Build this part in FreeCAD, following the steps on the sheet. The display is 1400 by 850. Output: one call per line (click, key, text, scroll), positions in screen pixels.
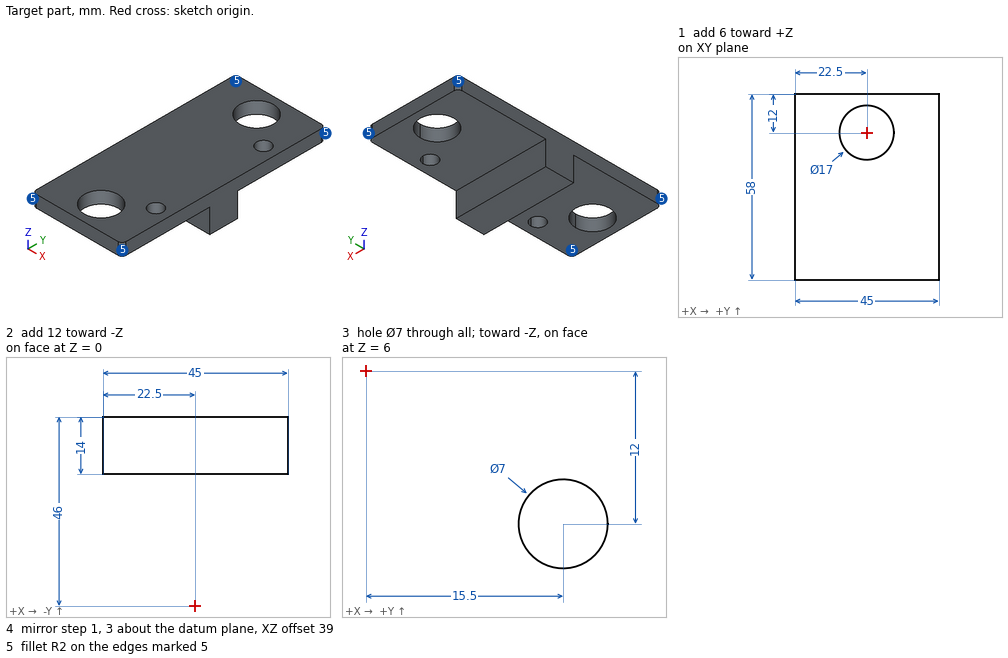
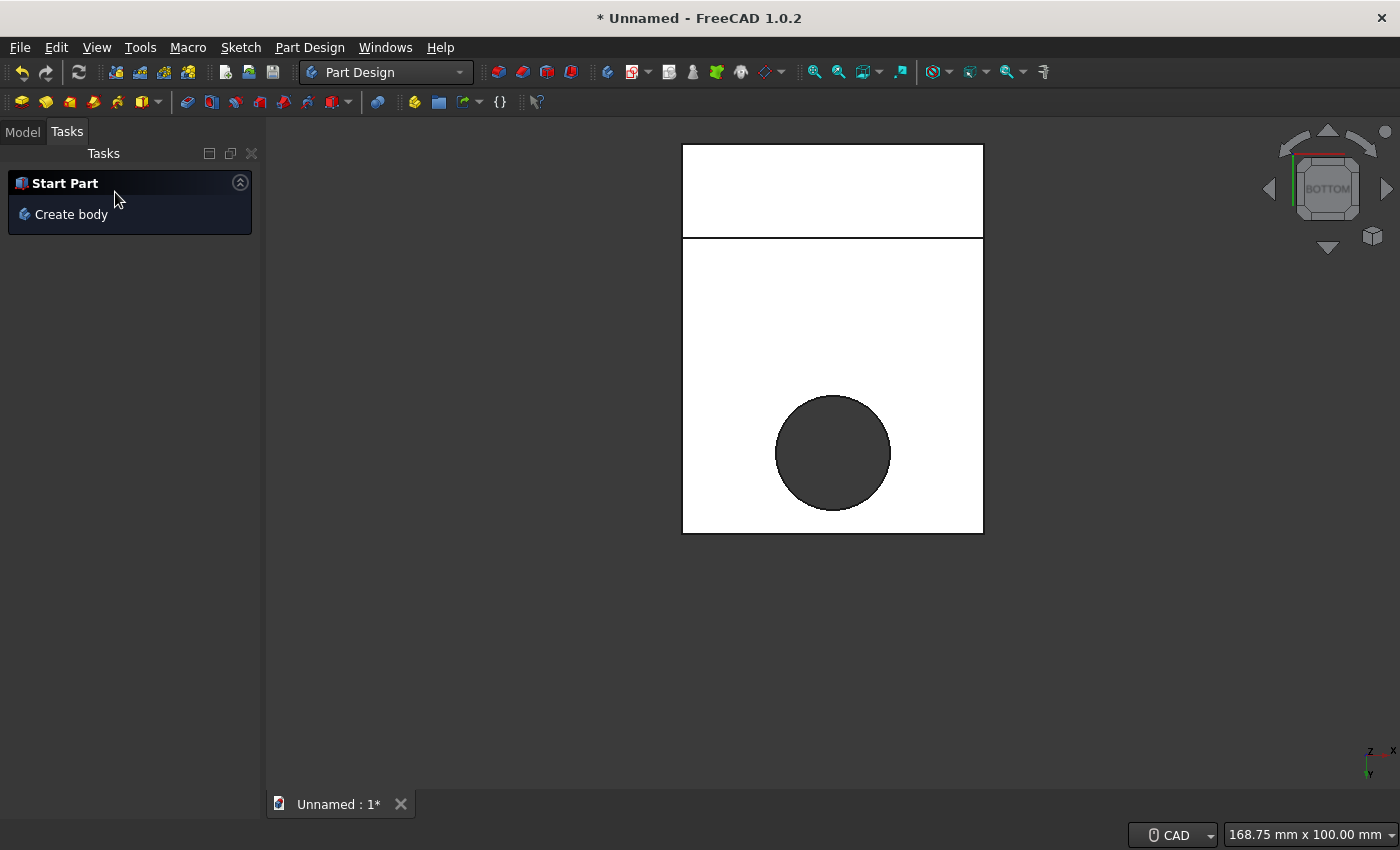
key(0)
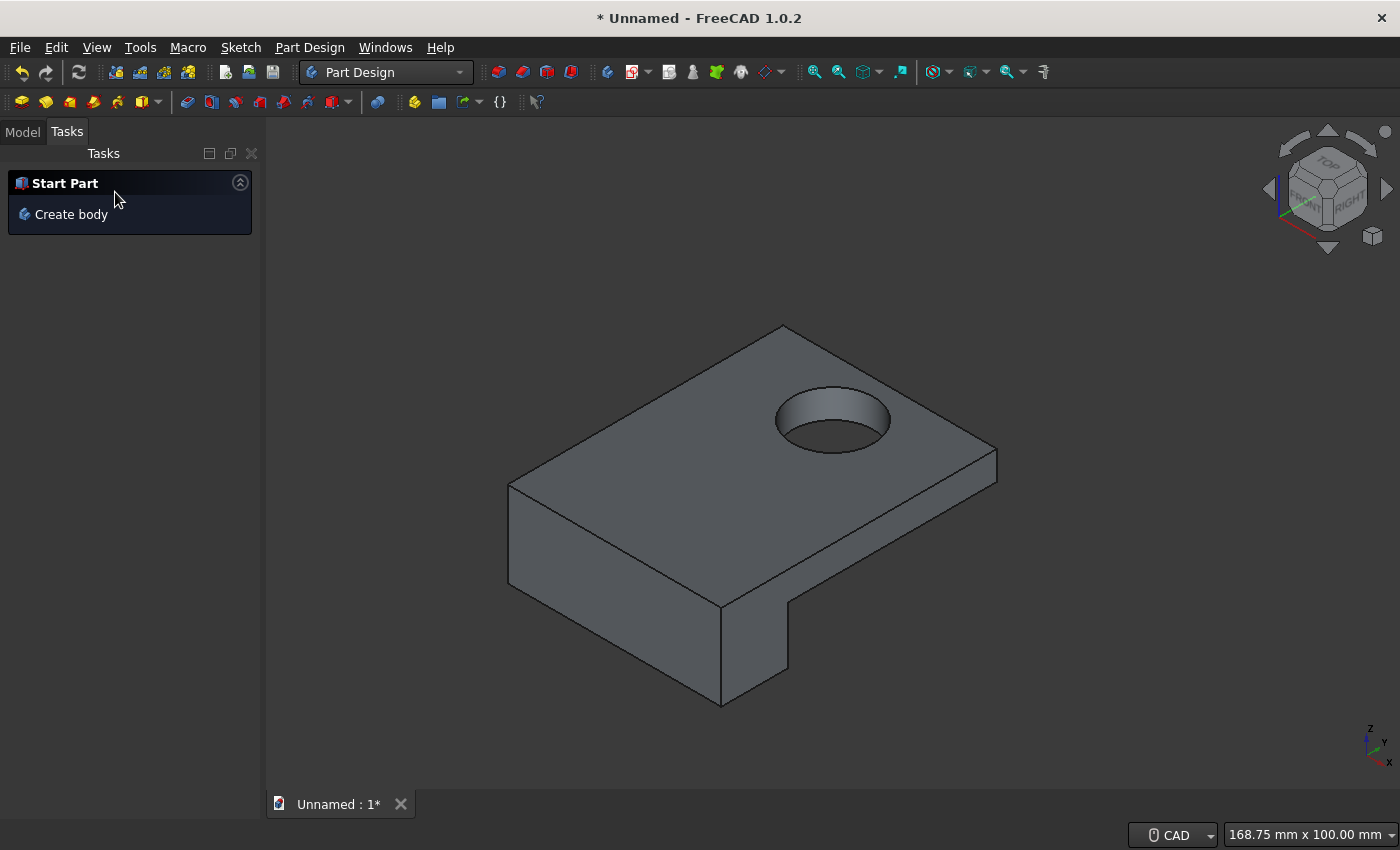
click(713, 488)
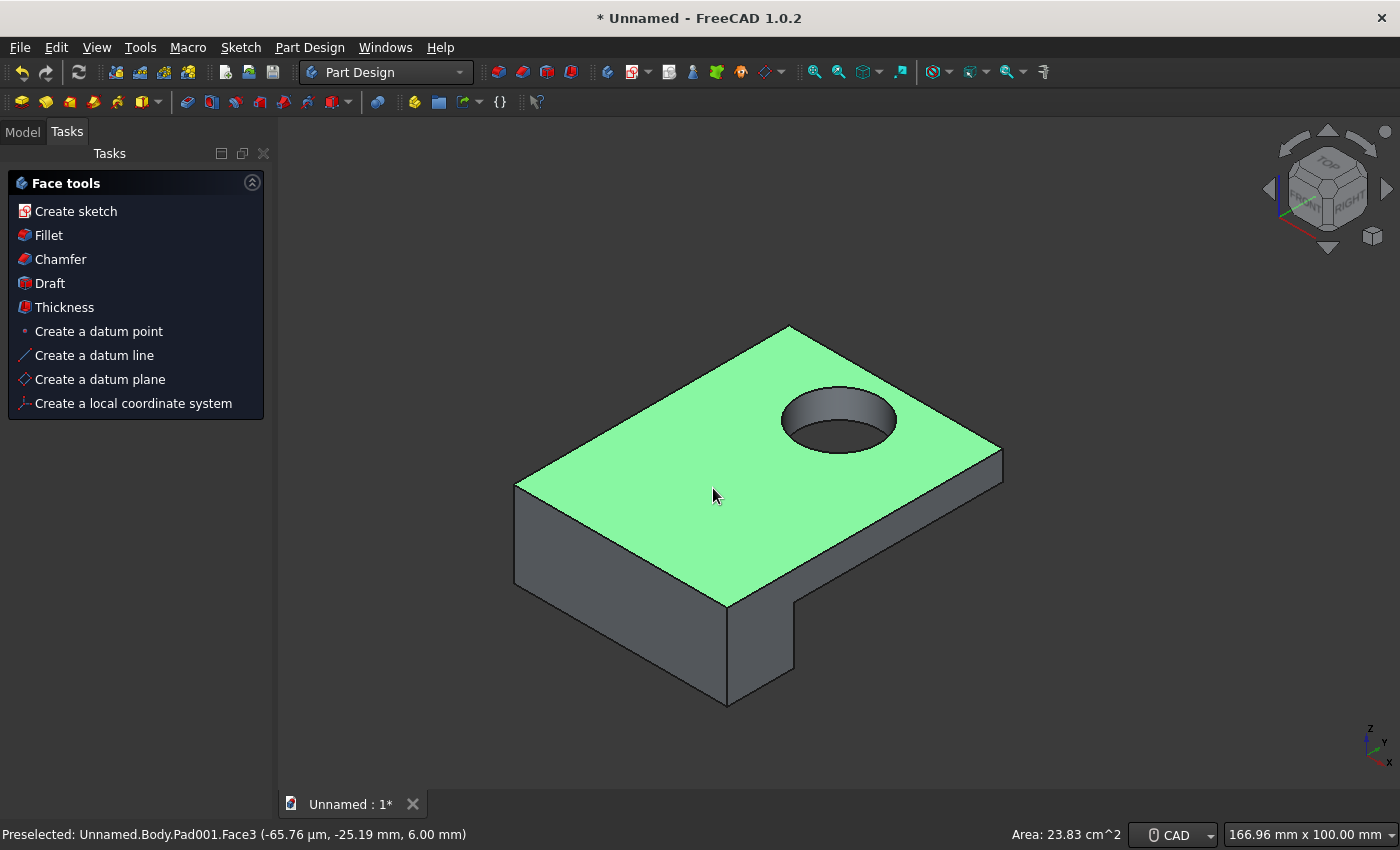
click(632, 72)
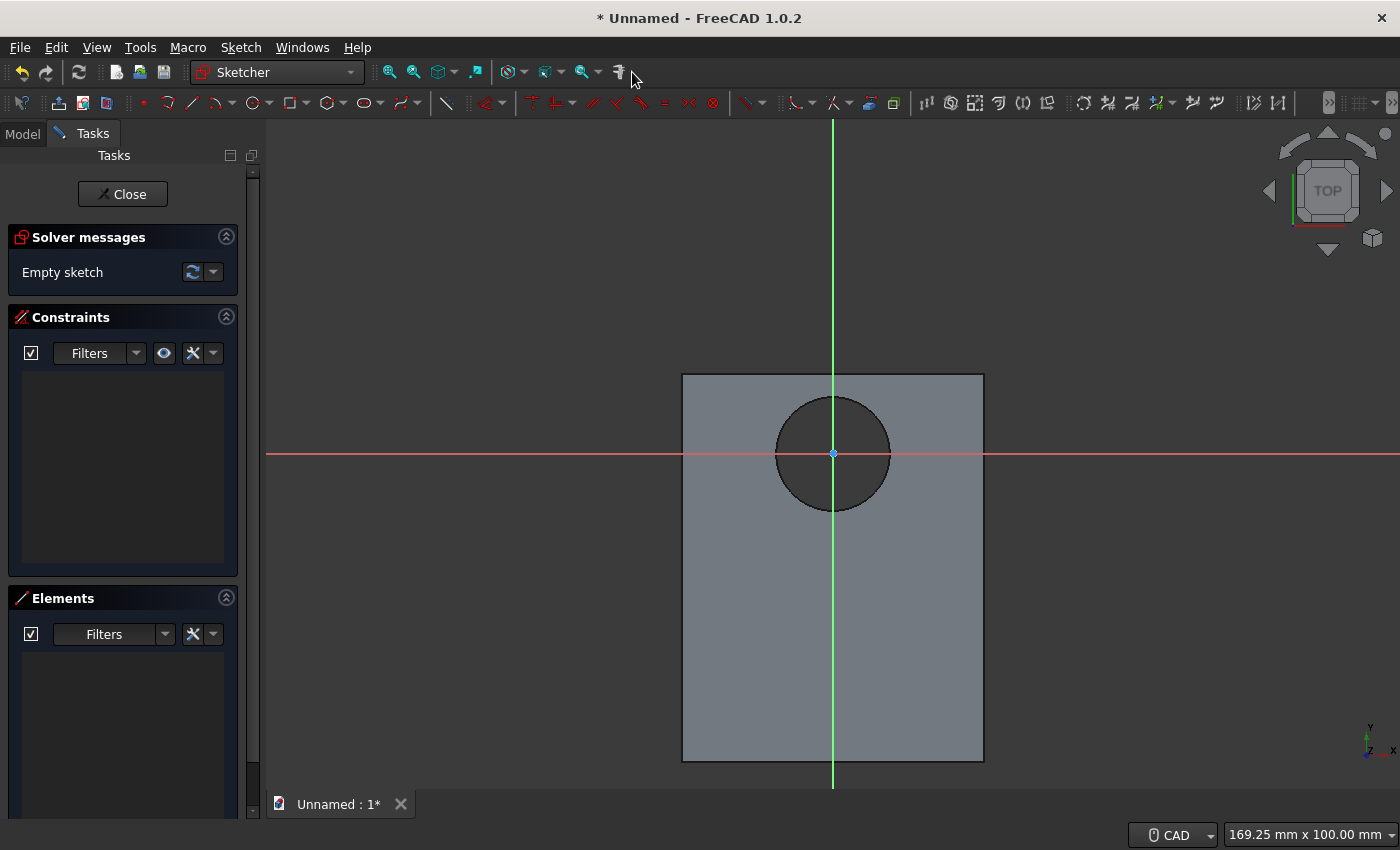
scroll(958, 544, up, 11)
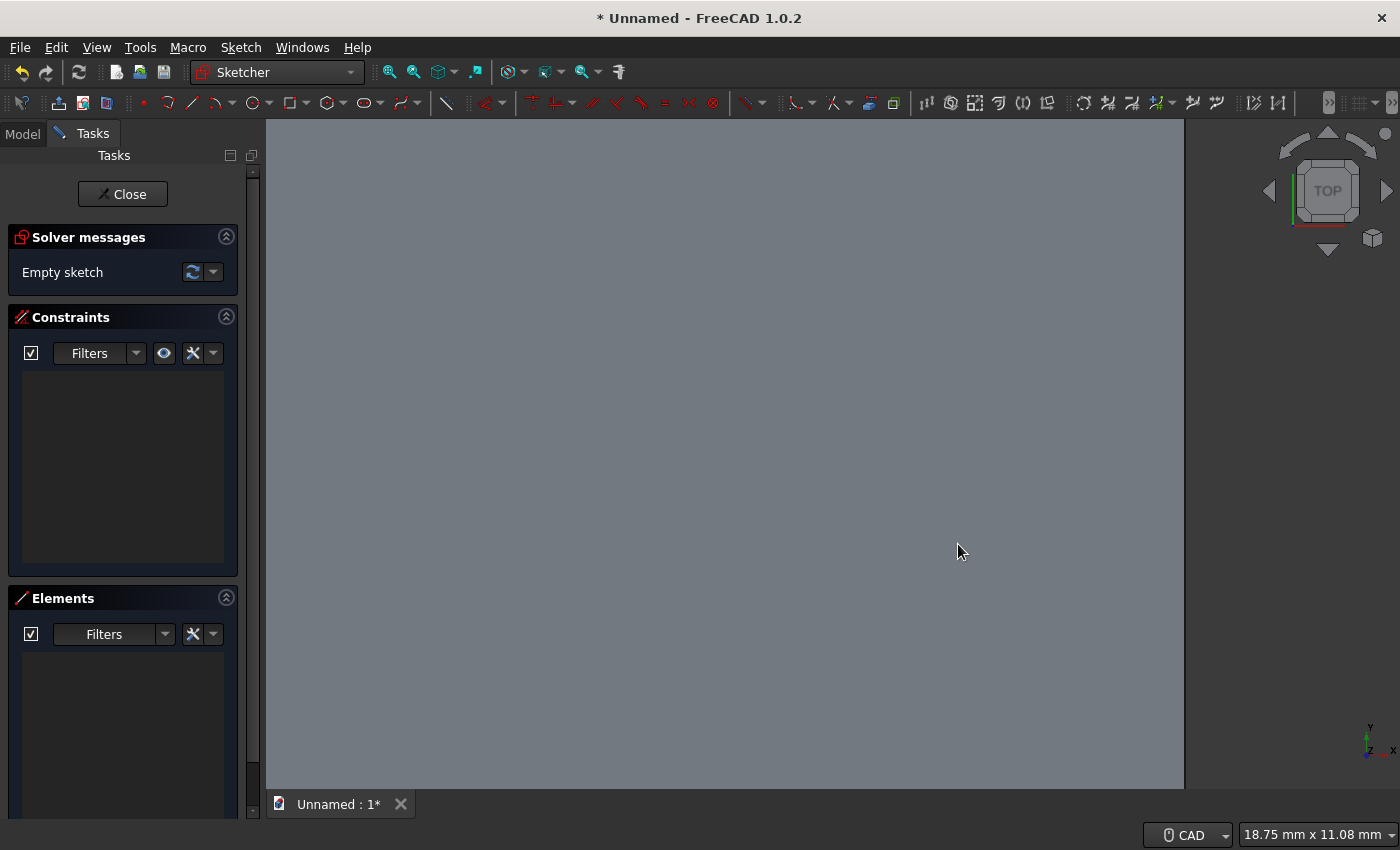
click(254, 104)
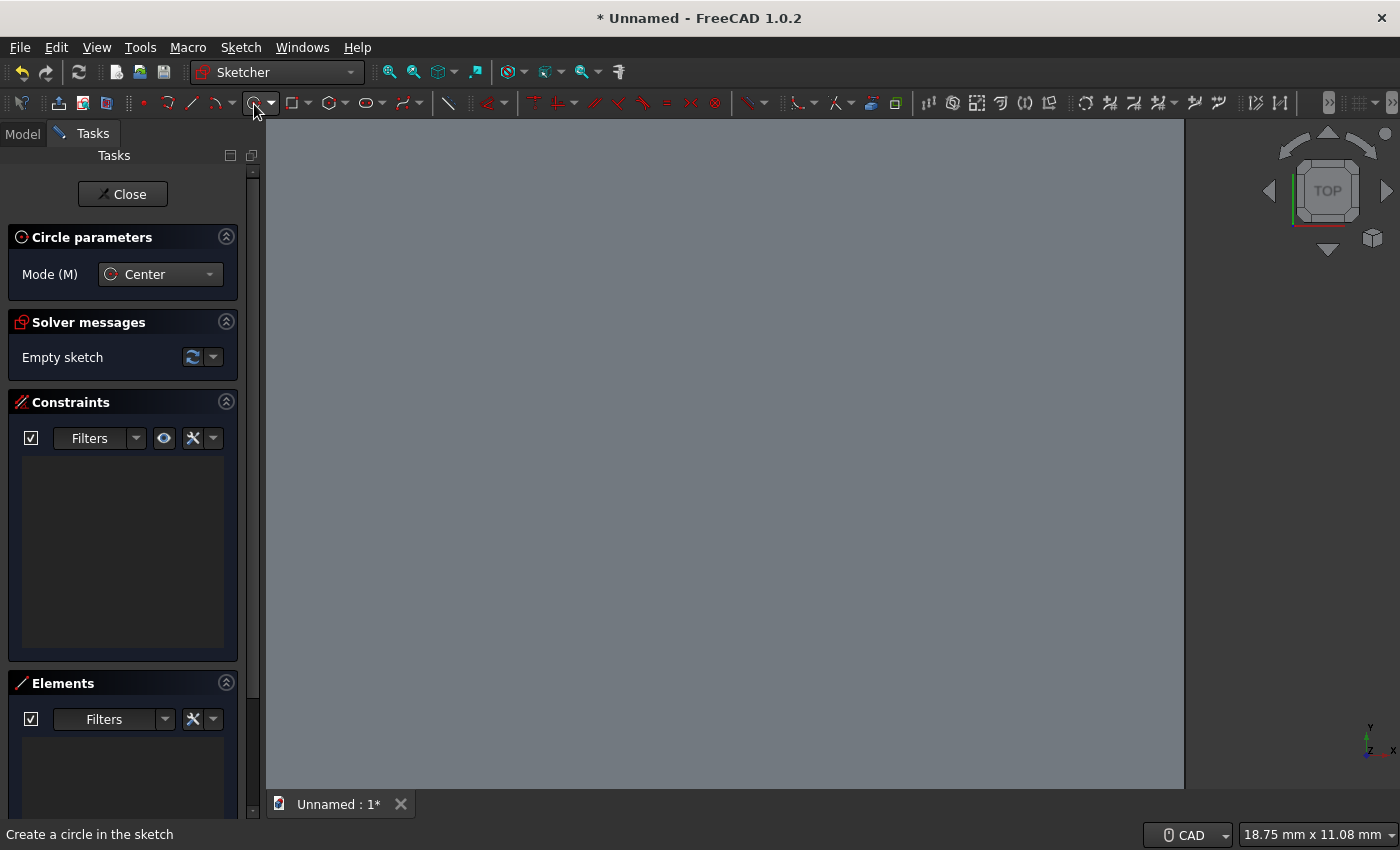
click(762, 452)
click(912, 303)
key(Escape)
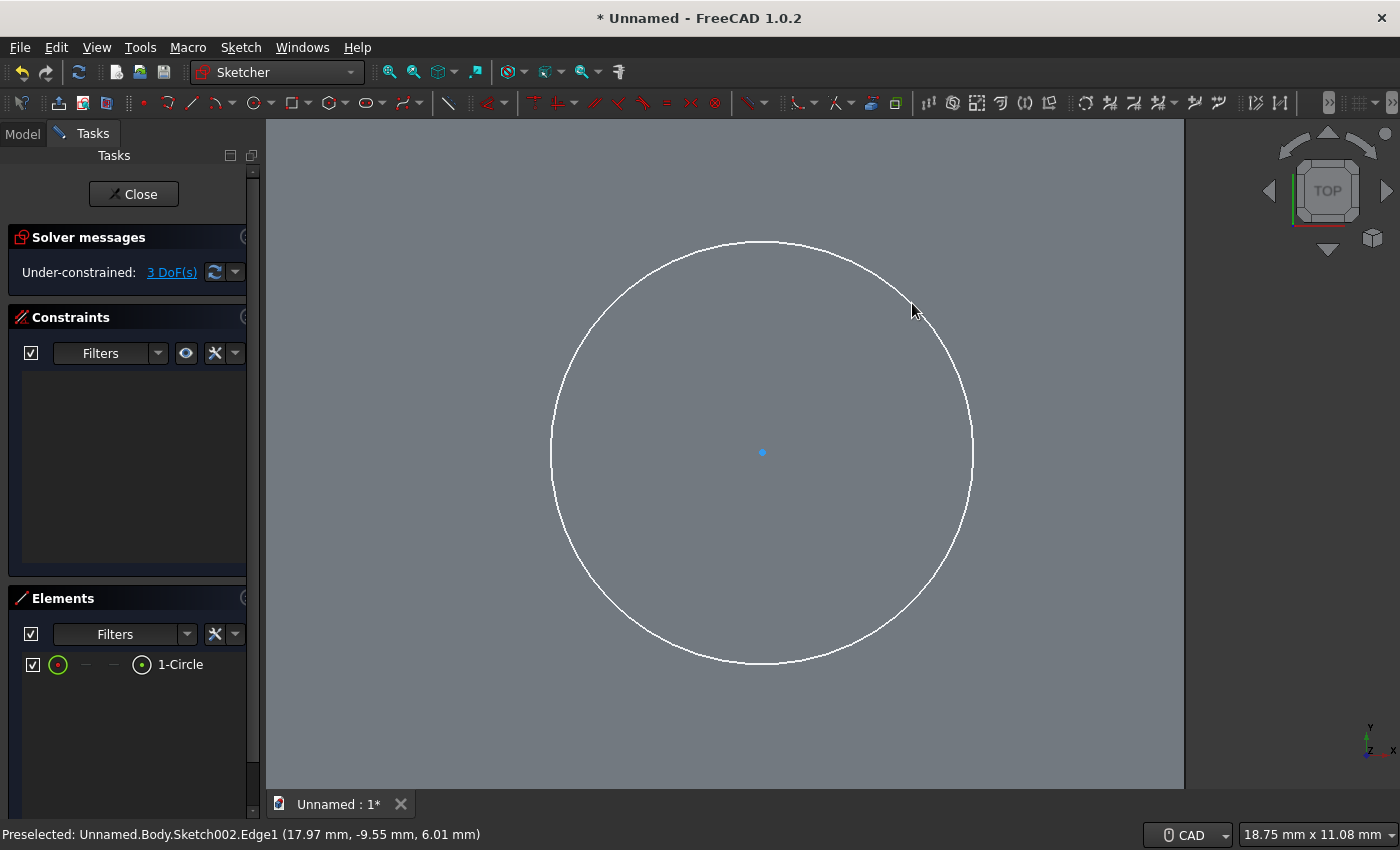
click(488, 104)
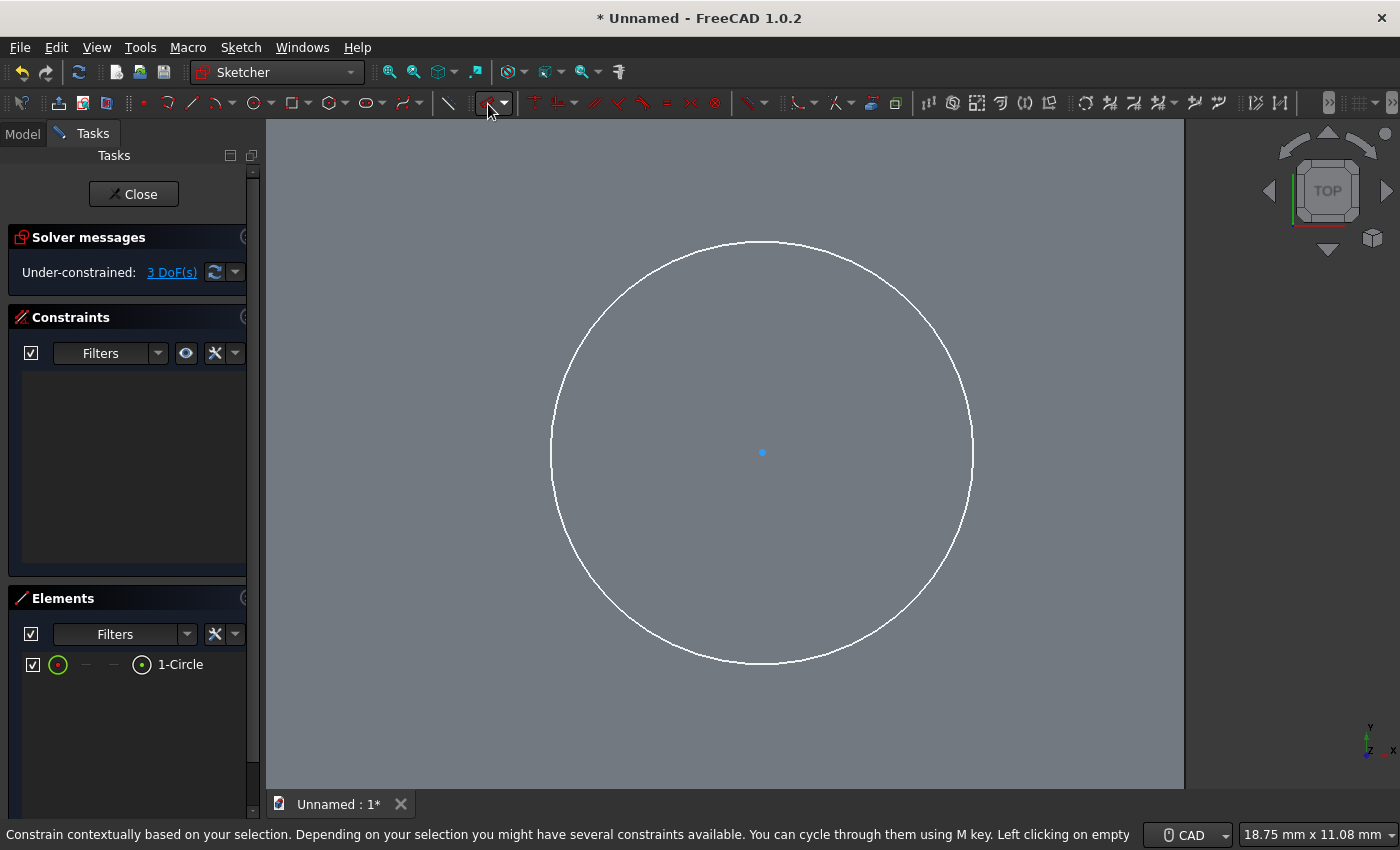
click(911, 303)
click(934, 280)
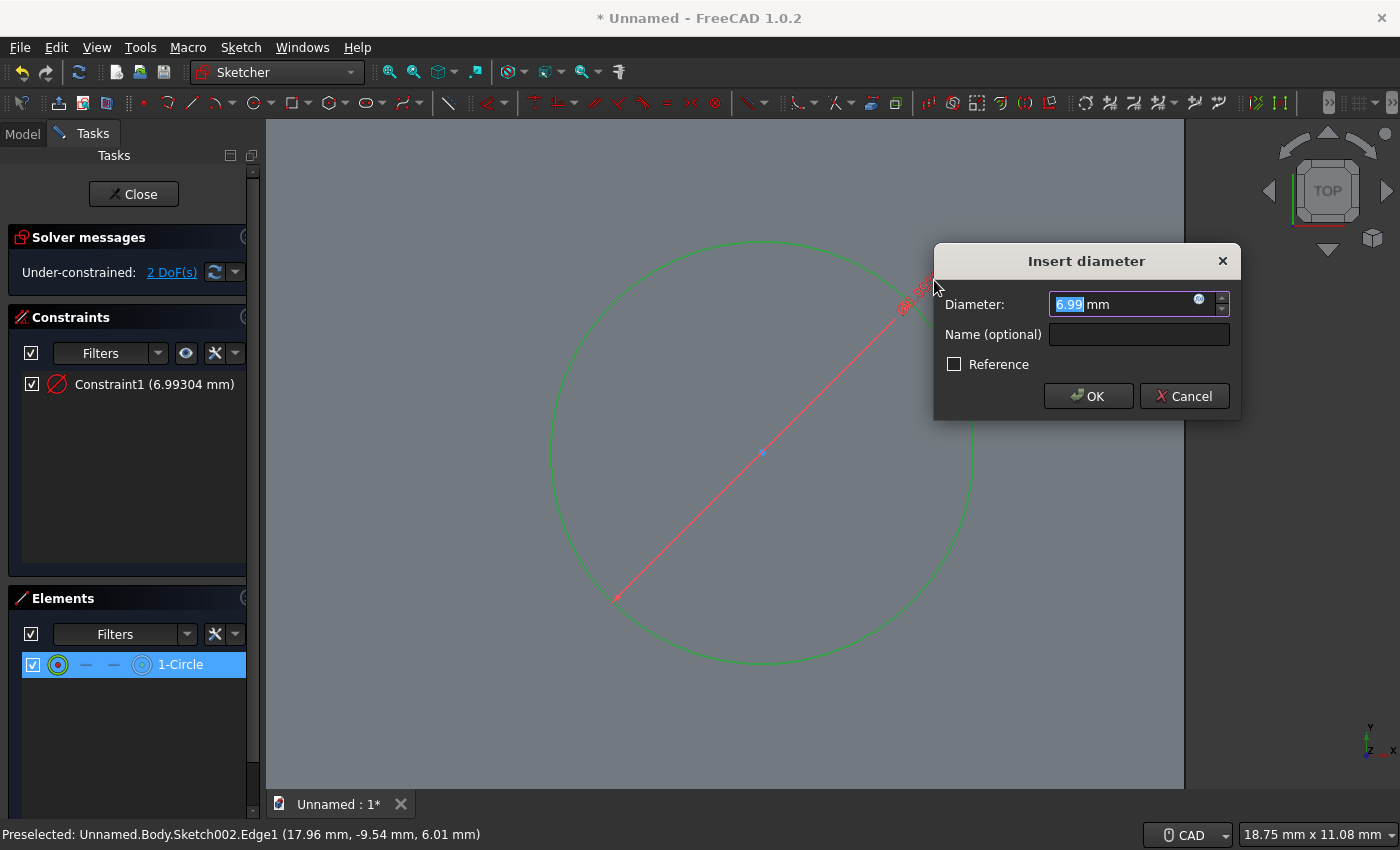
text(7)
key(Return)